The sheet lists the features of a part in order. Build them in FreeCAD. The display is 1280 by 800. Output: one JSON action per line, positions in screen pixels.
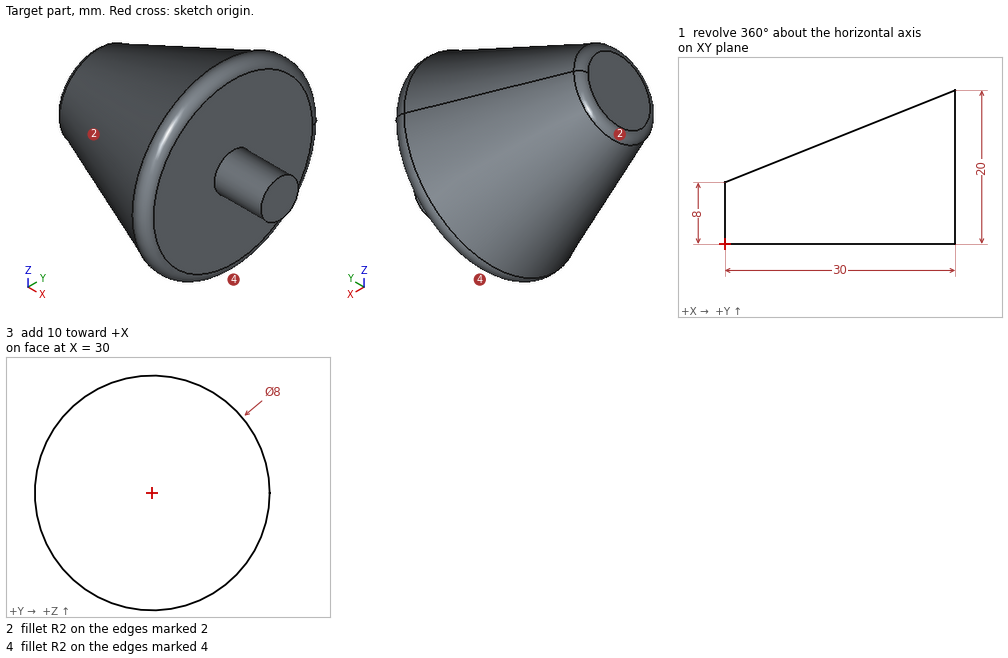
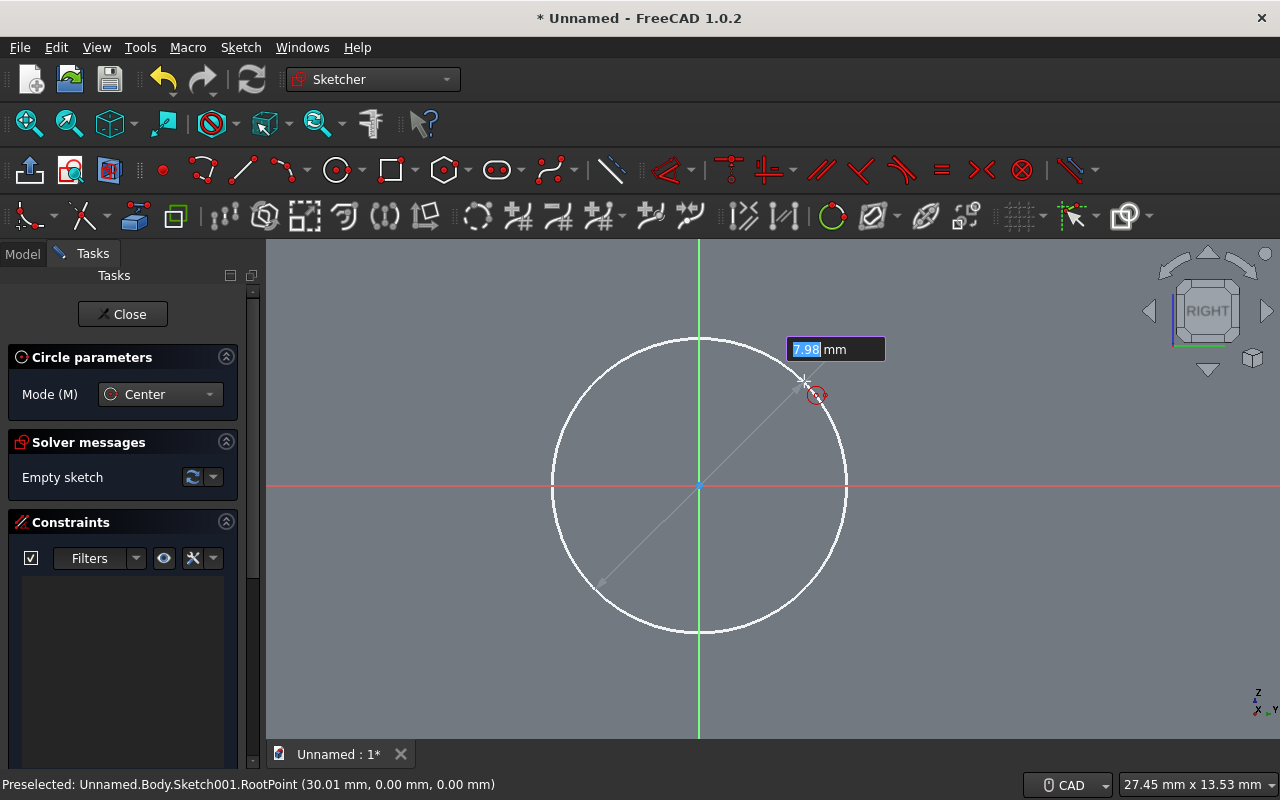
{"action": "type", "text": "8"}
{"action": "key", "text": "Return"}
{"action": "key", "text": "Escape"}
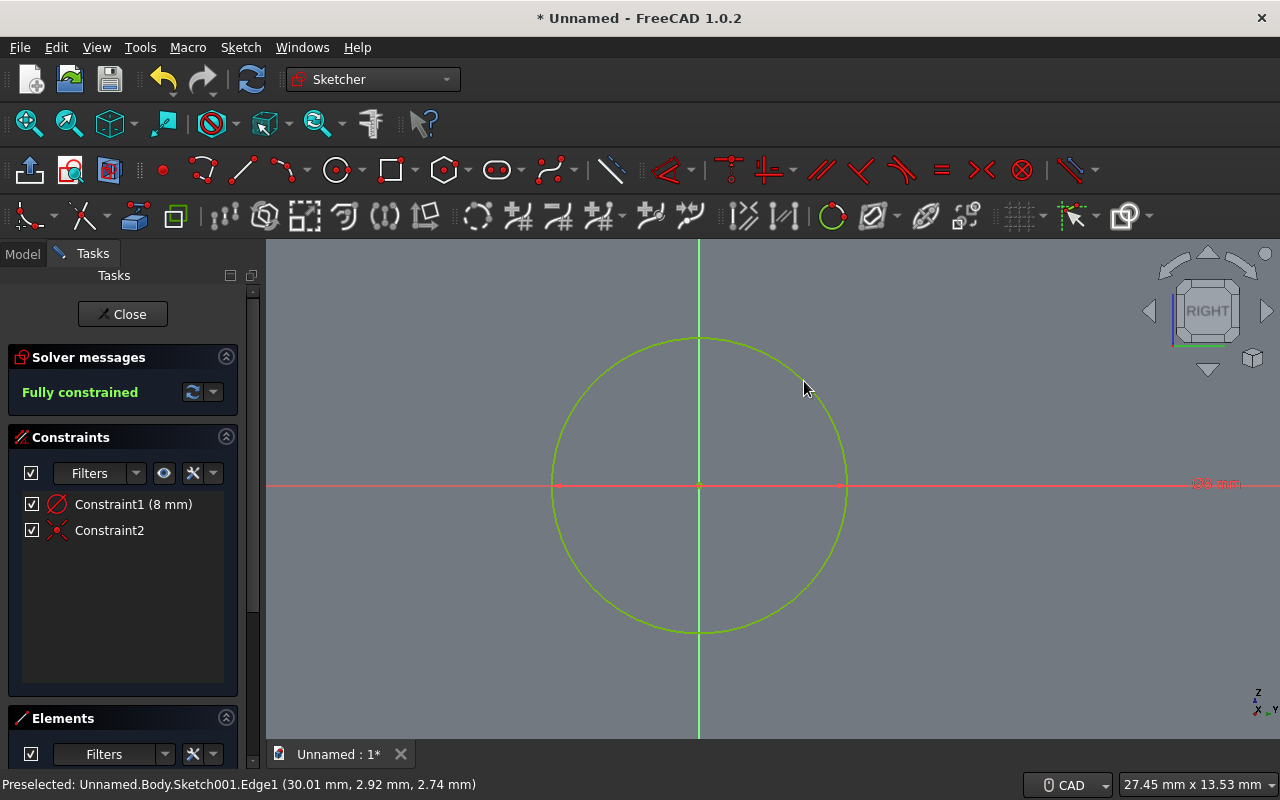
{"action": "left_click", "coordinate": [123, 314]}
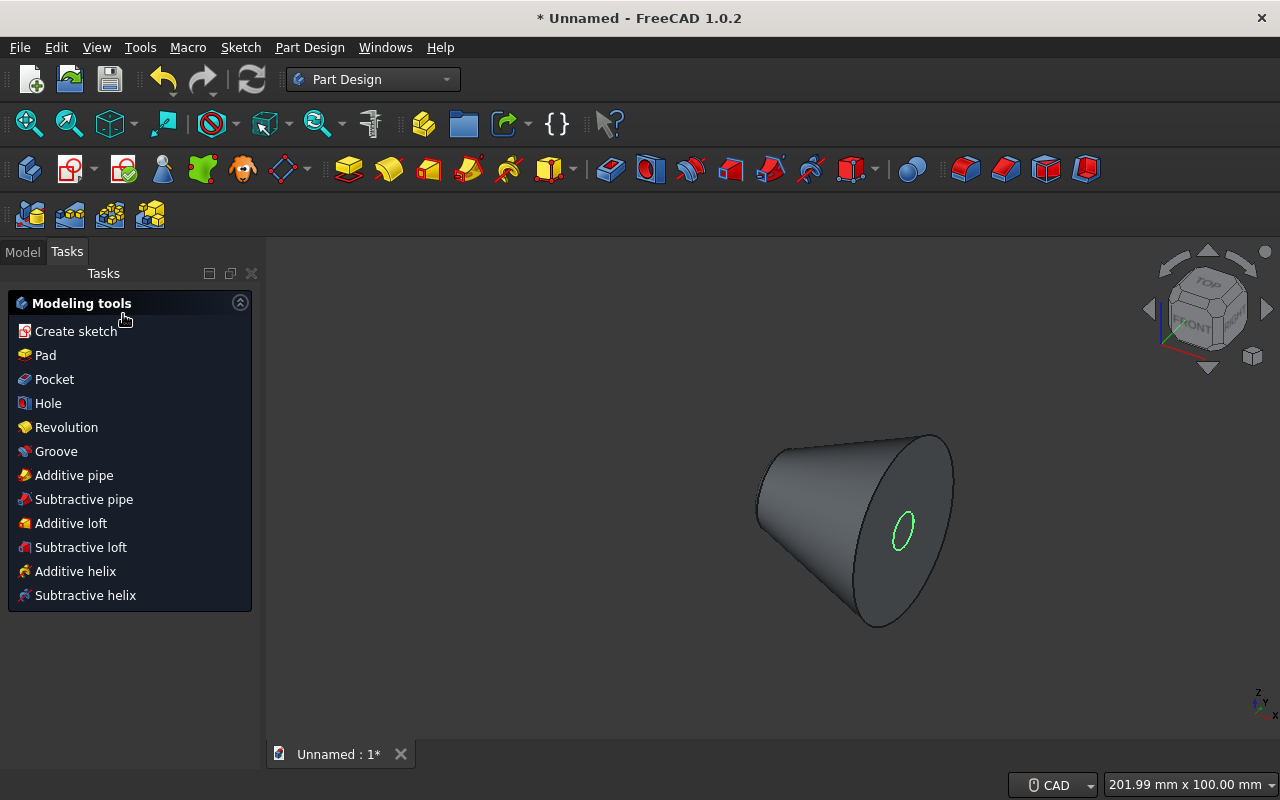
{"action": "left_click", "coordinate": [350, 170]}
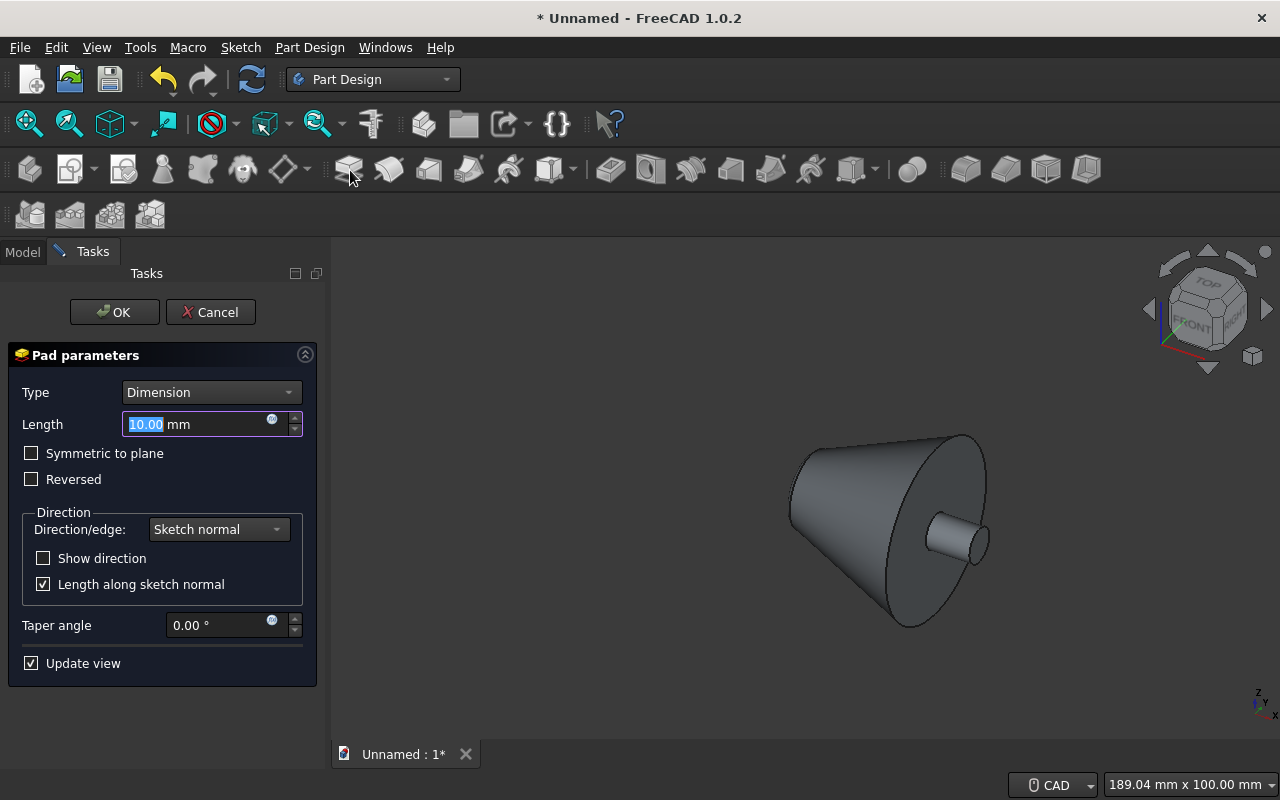
{"action": "type", "text": "10"}
{"action": "key", "text": "Tab"}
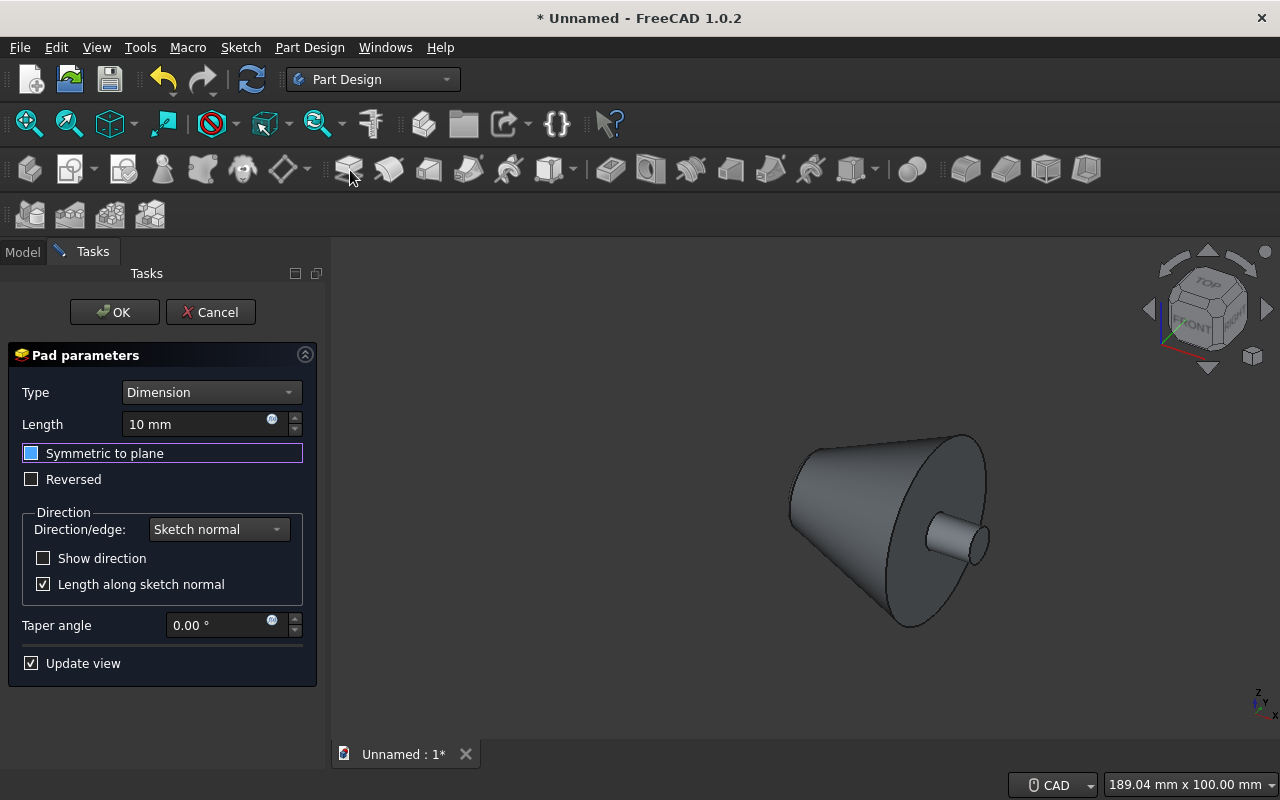
{"action": "left_click", "coordinate": [115, 312]}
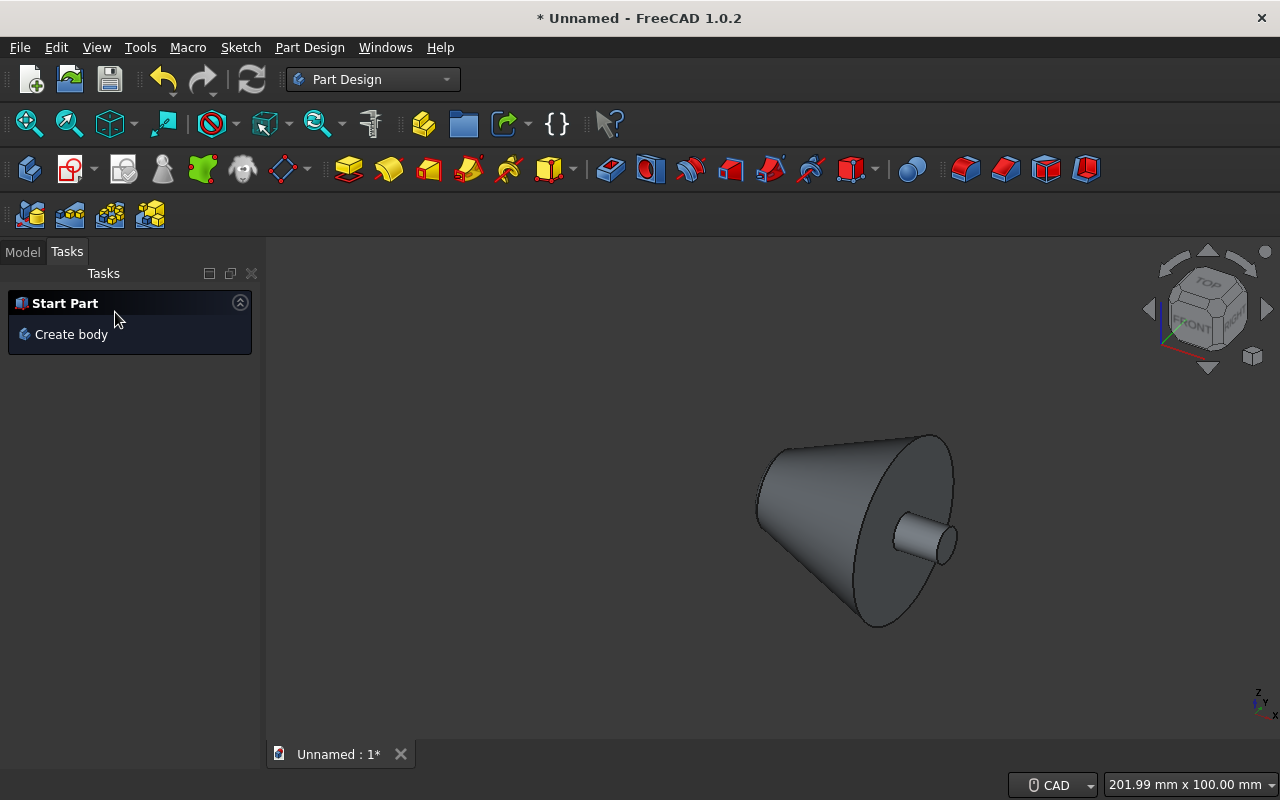
{"action": "left_click", "coordinate": [853, 580]}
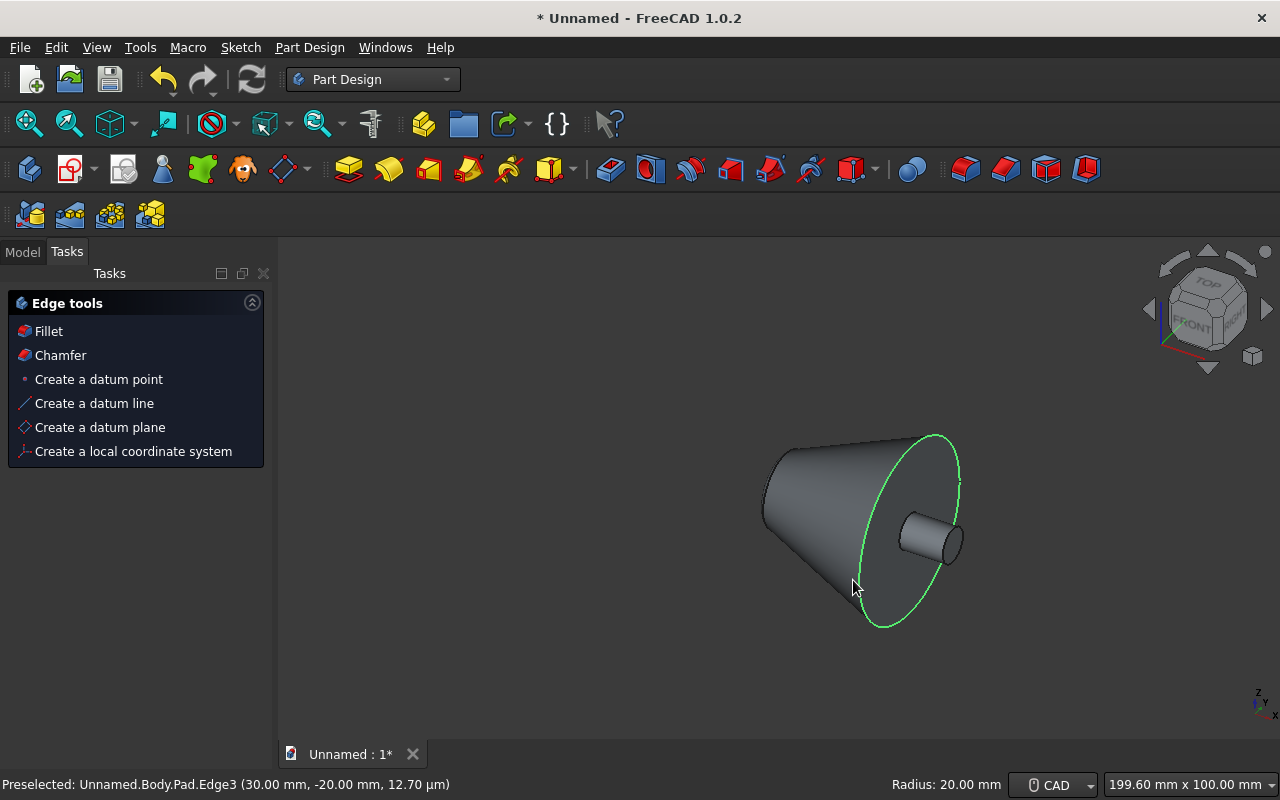
{"action": "left_click", "coordinate": [966, 170]}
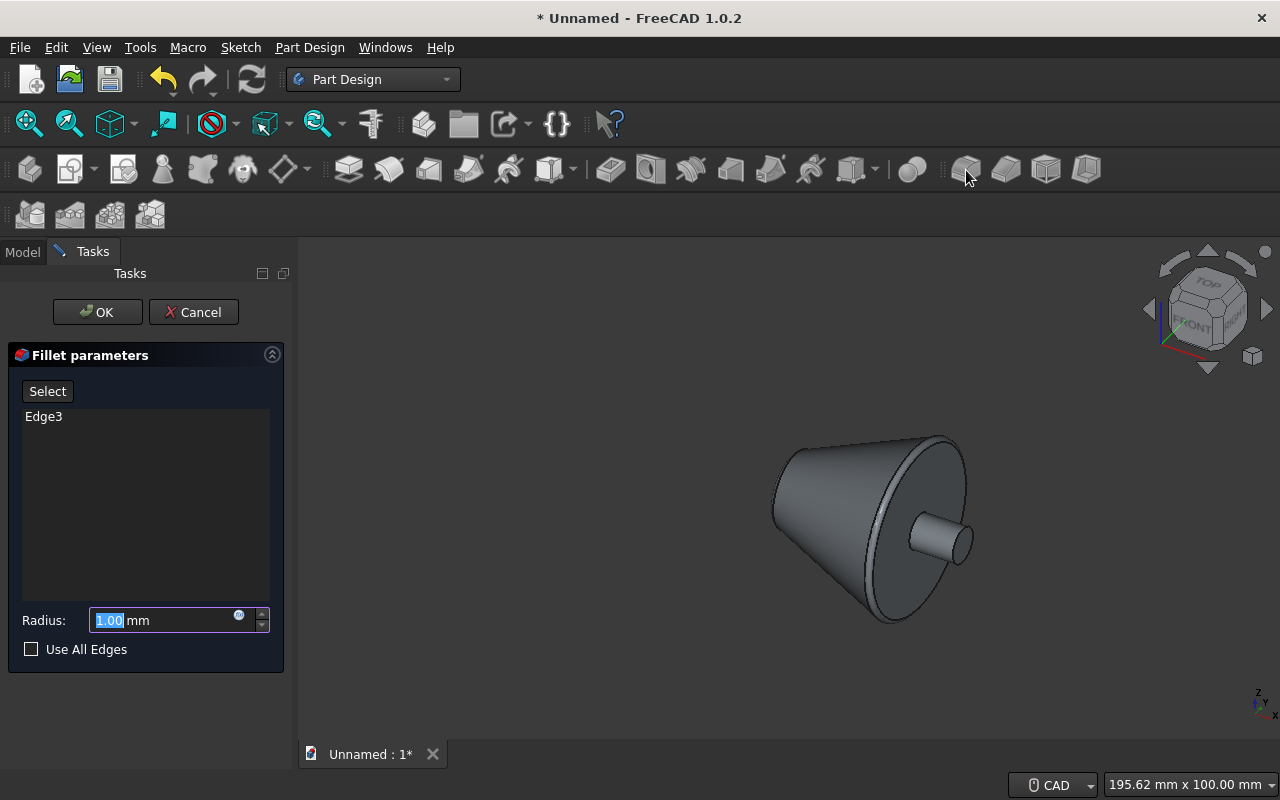
{"action": "type", "text": "2"}
{"action": "key", "text": "Tab"}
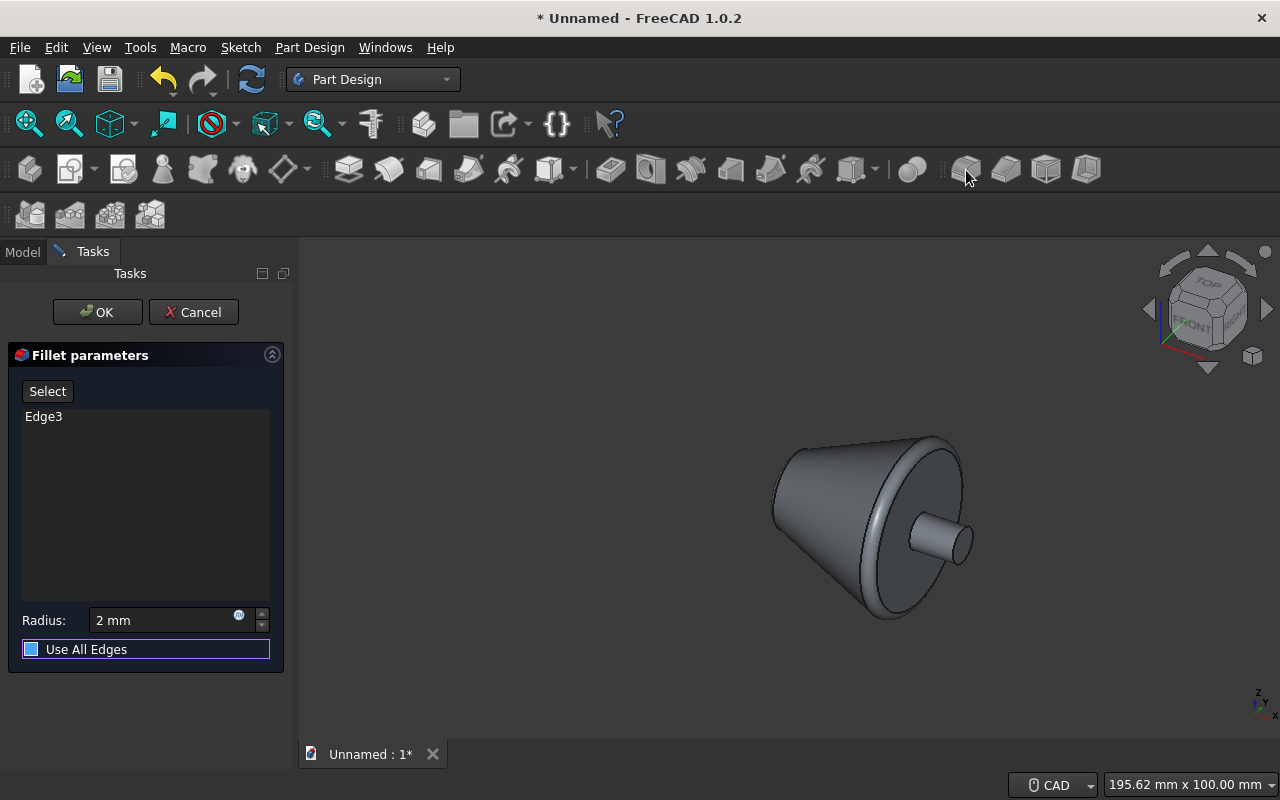
{"action": "left_click", "coordinate": [98, 312]}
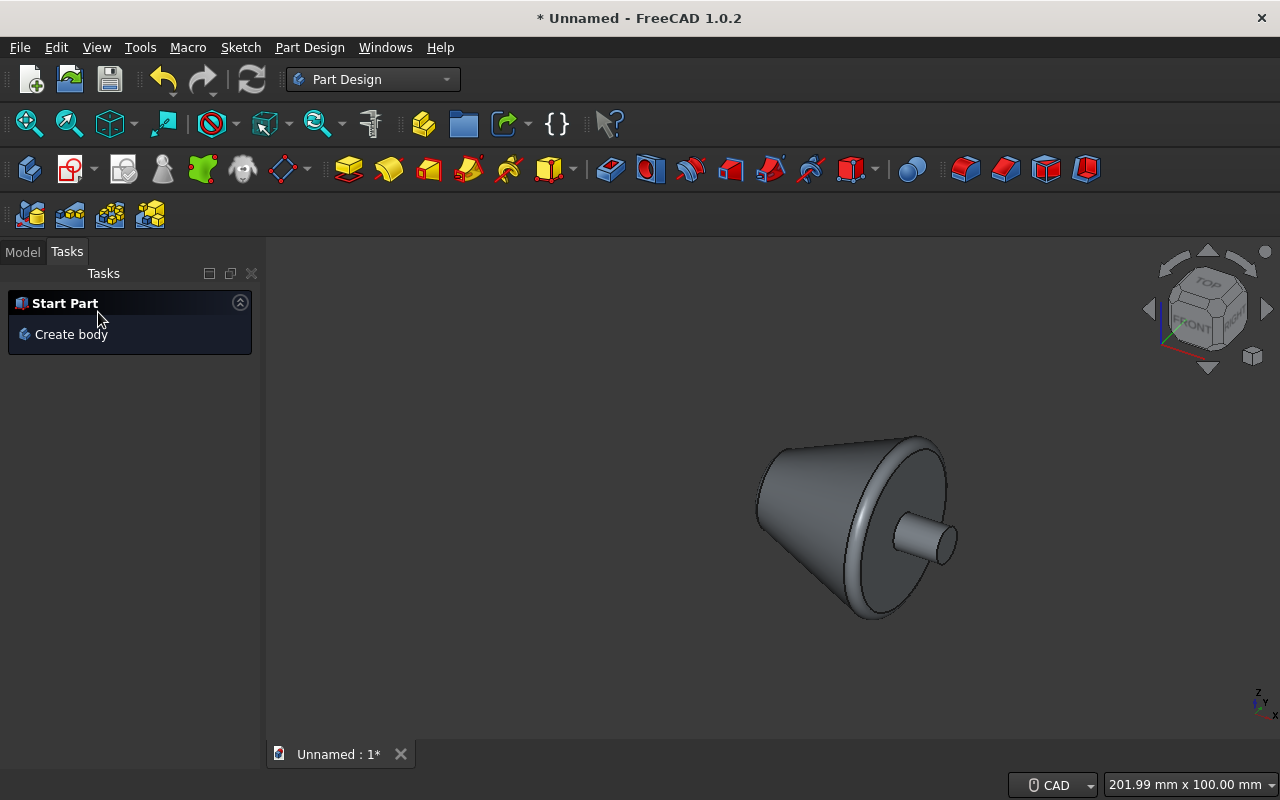
{"action": "key", "text": "0"}